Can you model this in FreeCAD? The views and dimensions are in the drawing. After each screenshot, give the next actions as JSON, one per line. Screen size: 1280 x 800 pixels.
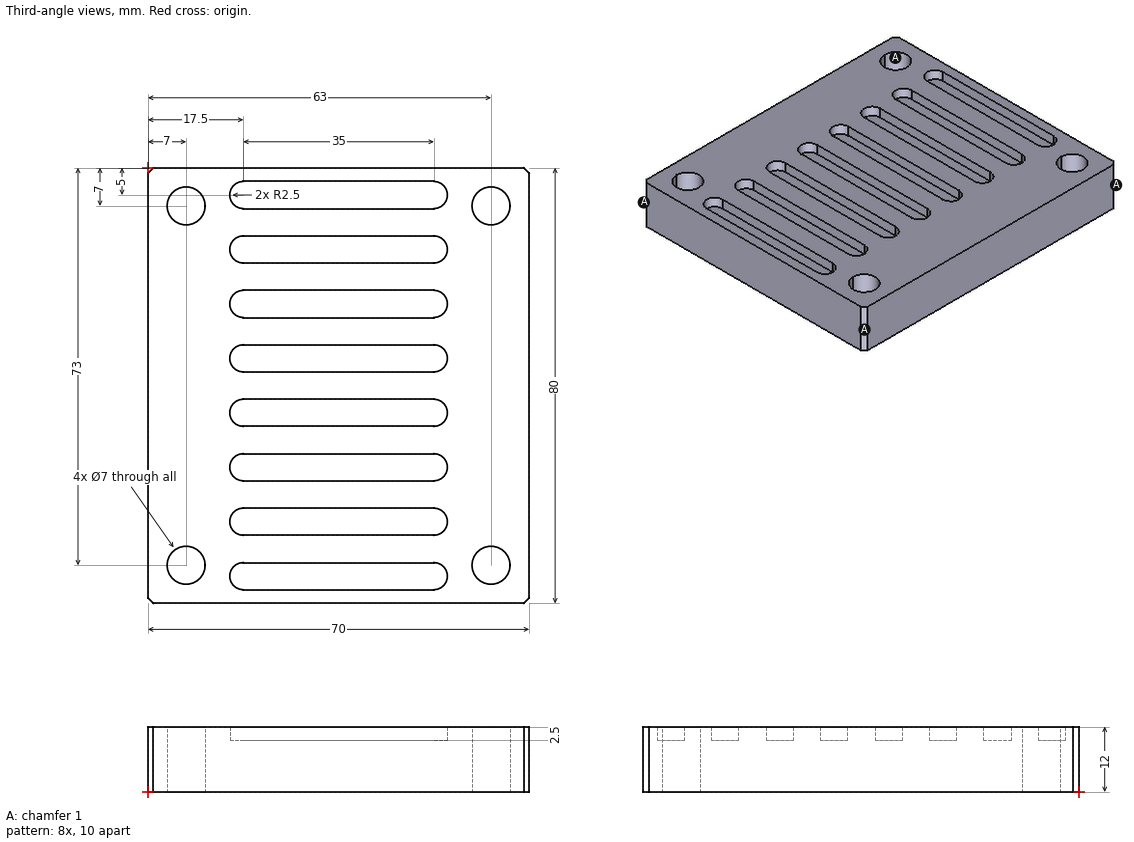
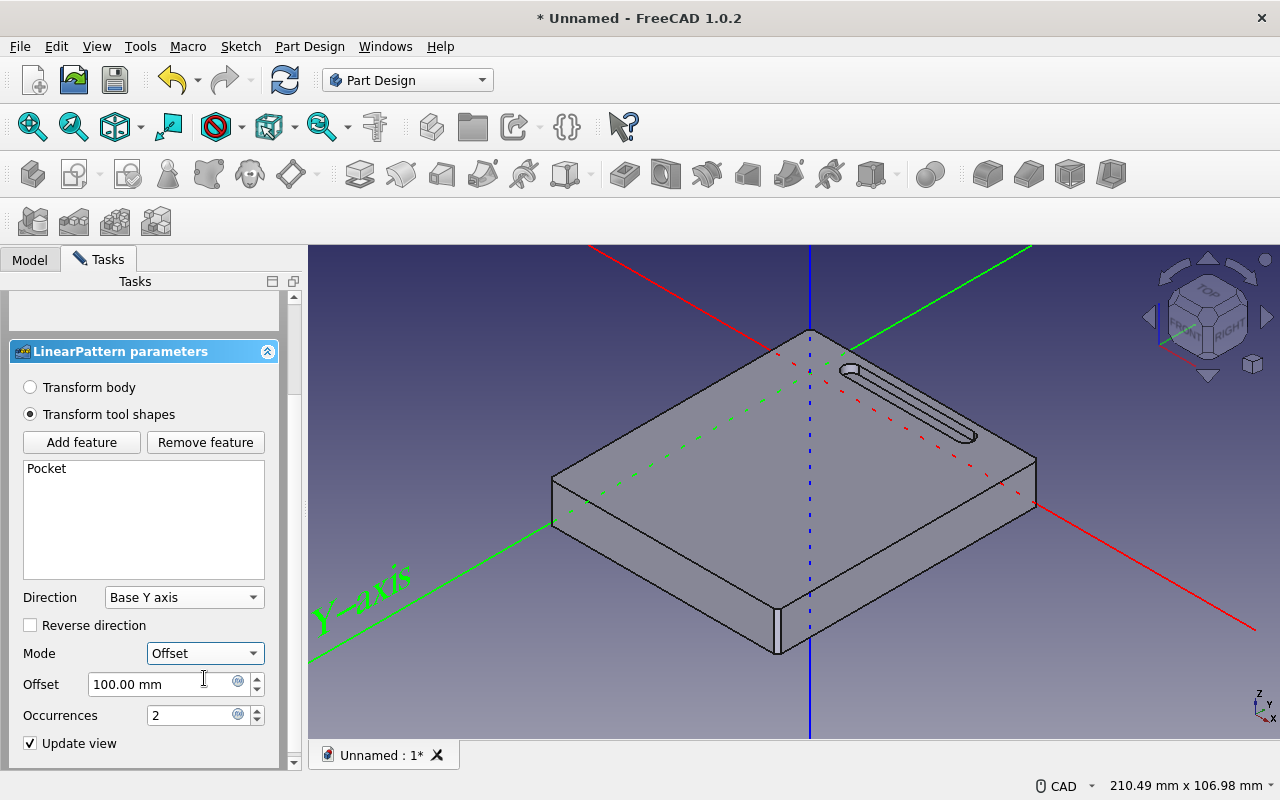
{"action": "triple_click", "coordinate": [170, 684]}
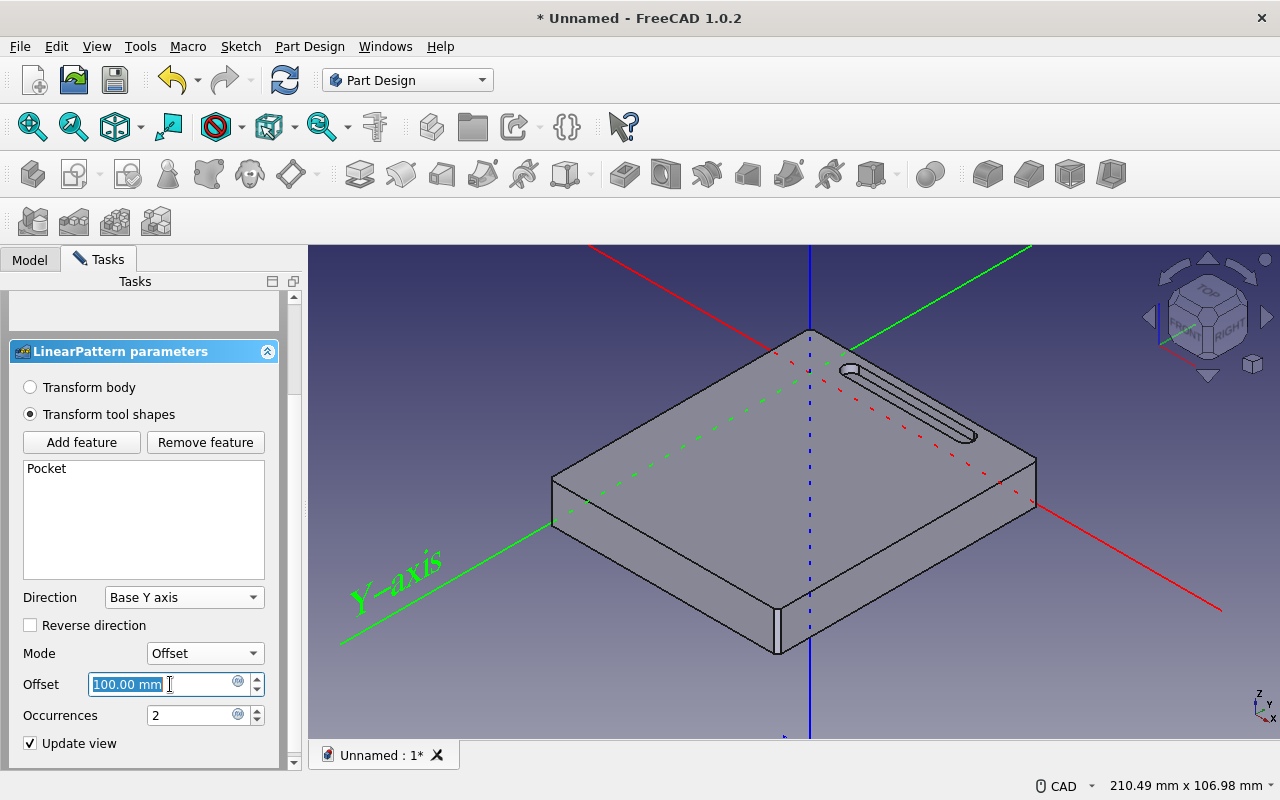
{"action": "type", "text": "10"}
{"action": "key", "text": "Tab"}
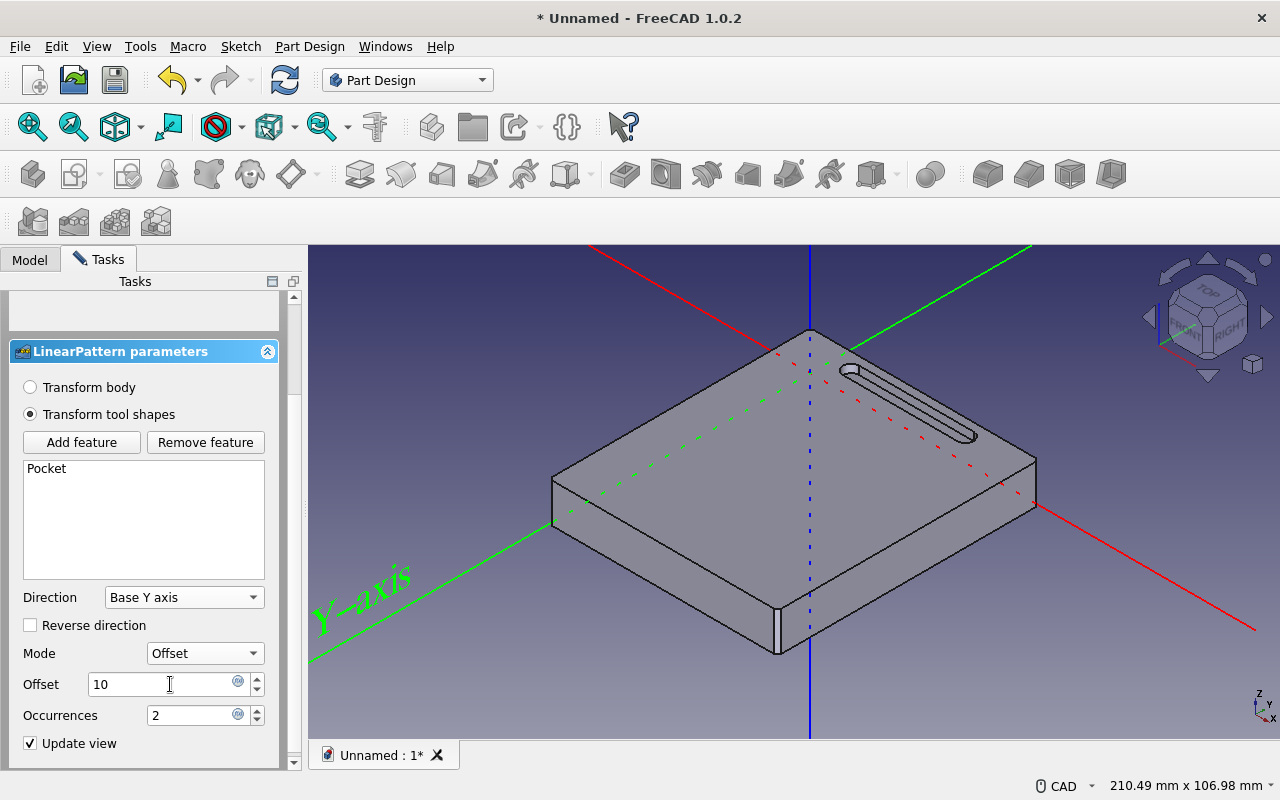
{"action": "triple_click", "coordinate": [199, 716]}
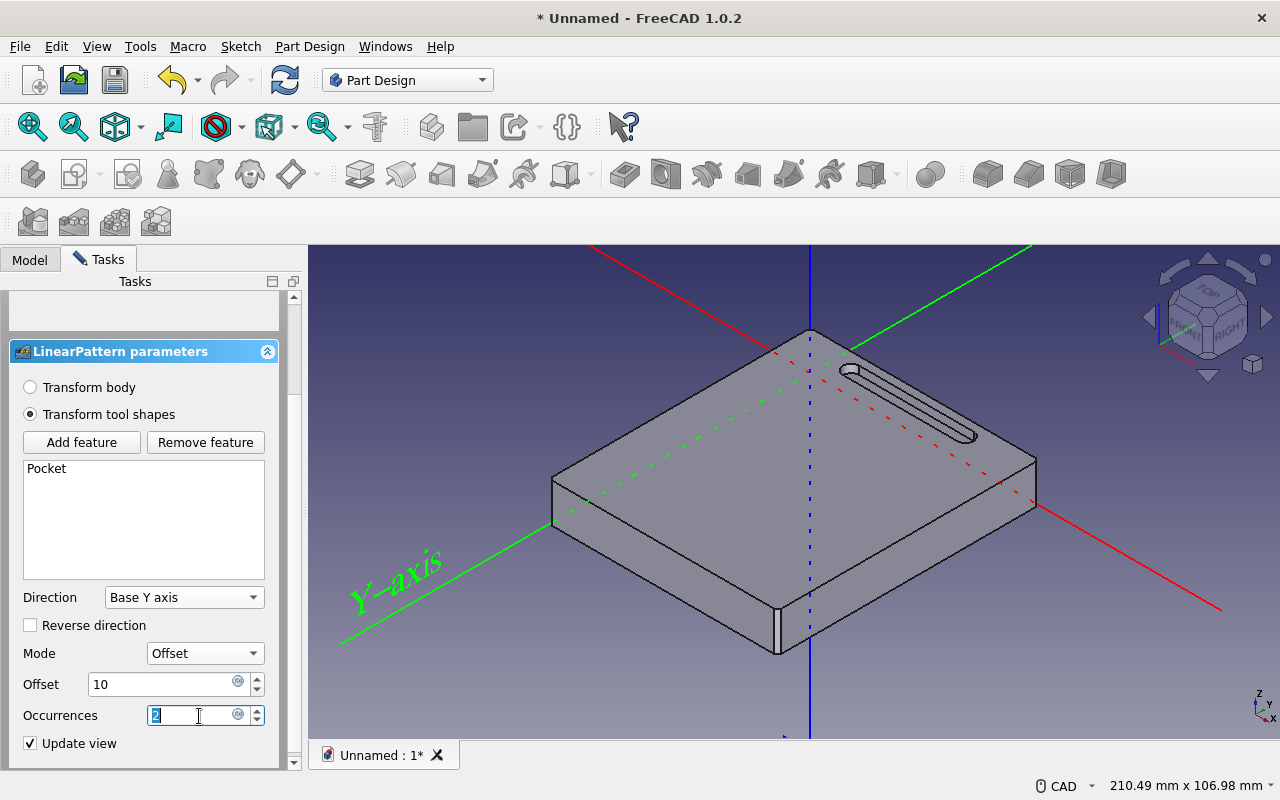
{"action": "type", "text": "8"}
{"action": "key", "text": "Tab"}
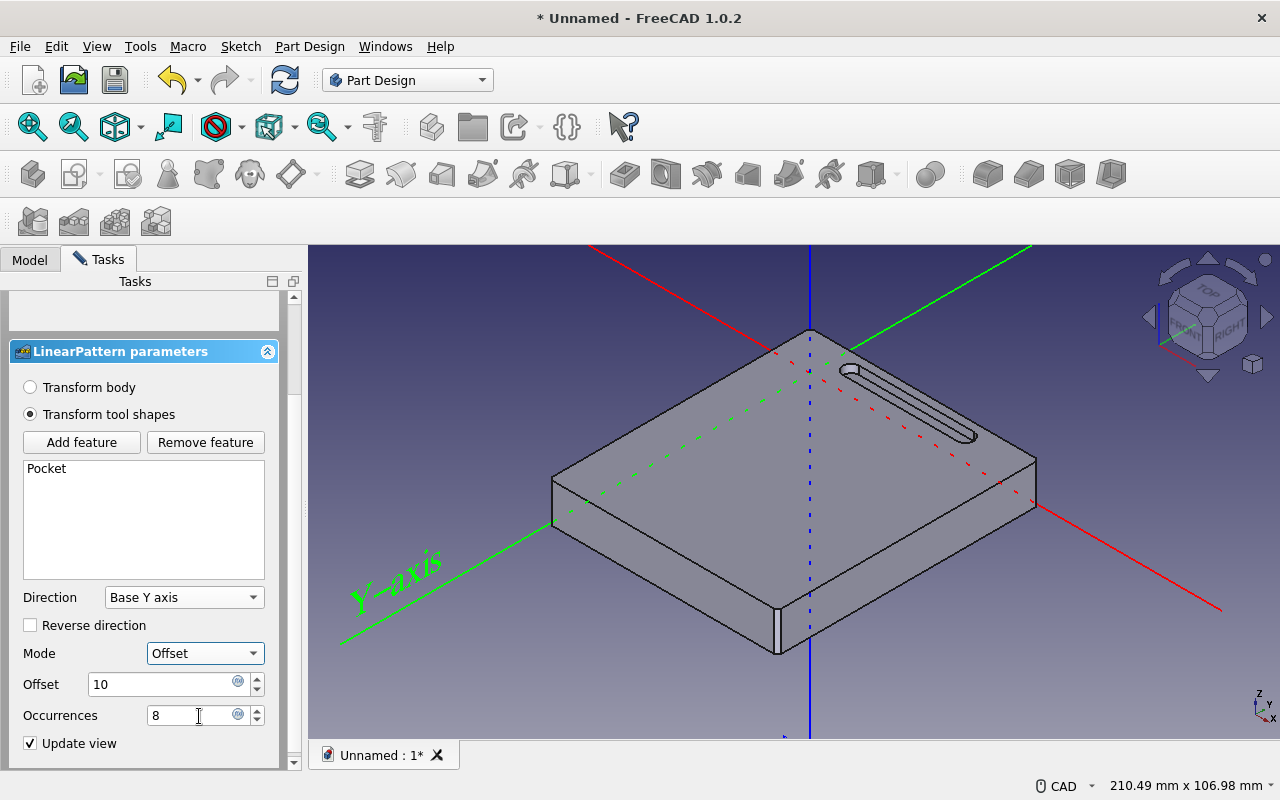
{"action": "left_click", "coordinate": [31, 625]}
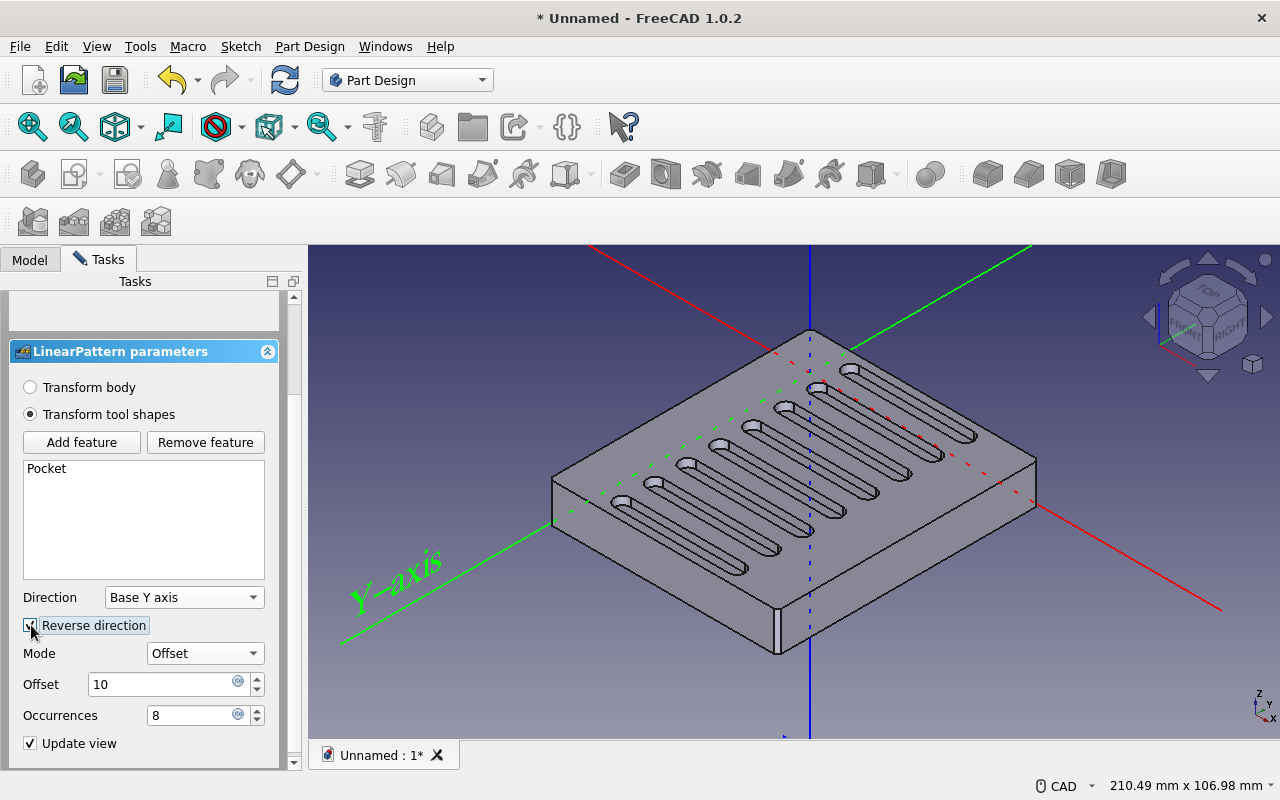
{"action": "scroll", "coordinate": [294, 530], "scroll_direction": "up", "scroll_amount": 3}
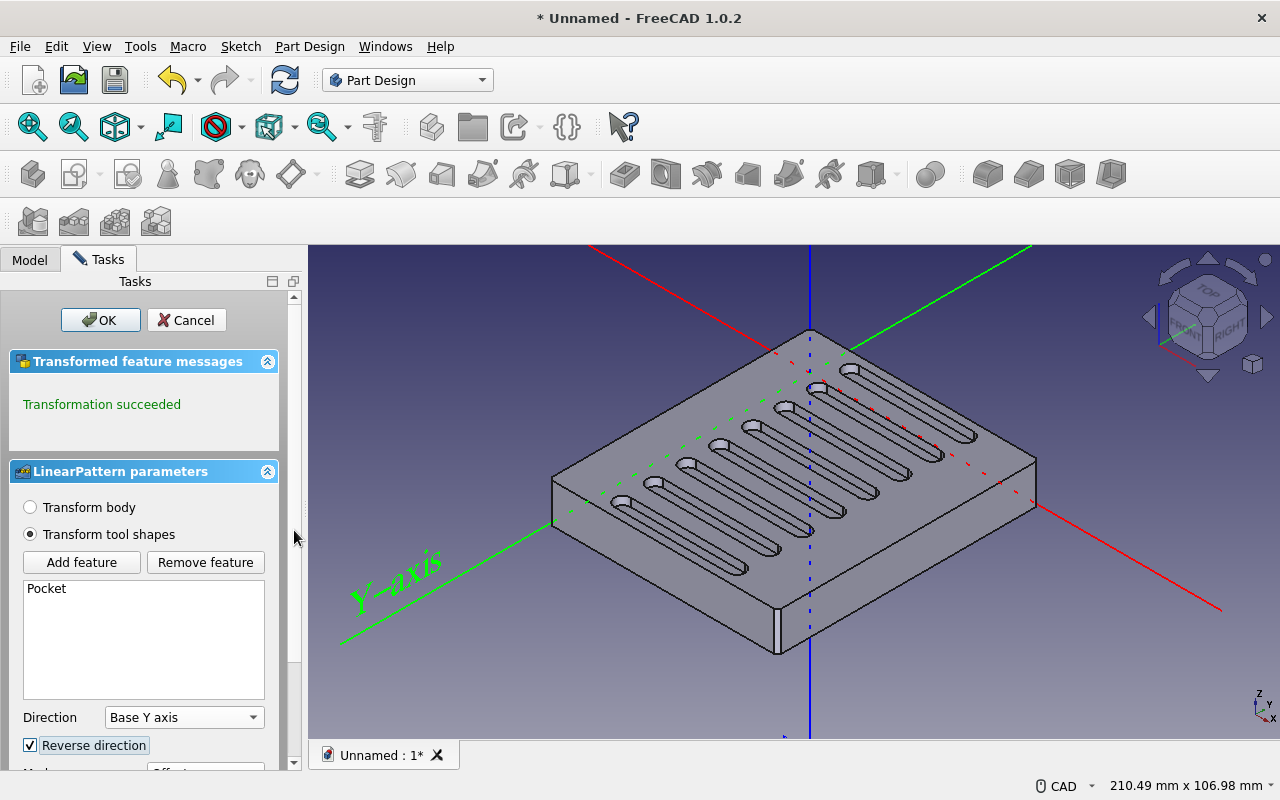
{"action": "left_click", "coordinate": [101, 320]}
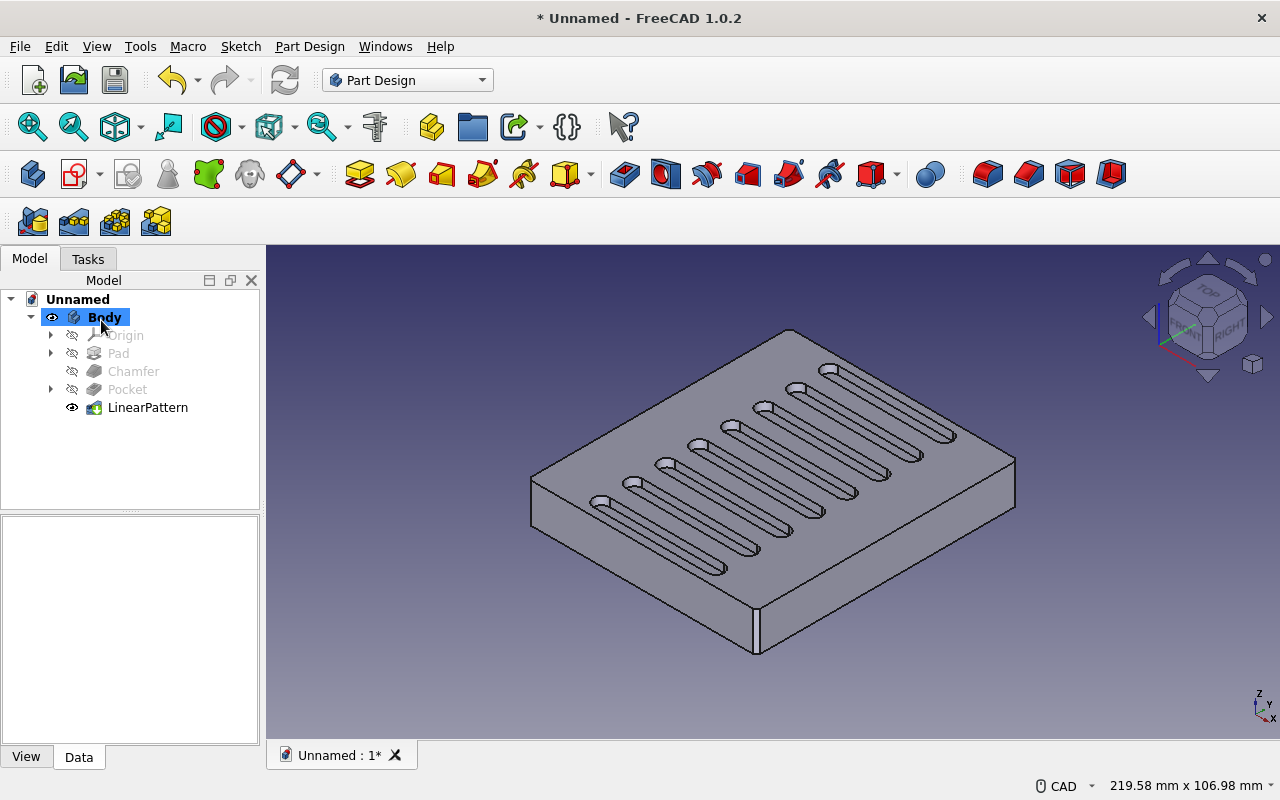
{"action": "left_click", "coordinate": [74, 174]}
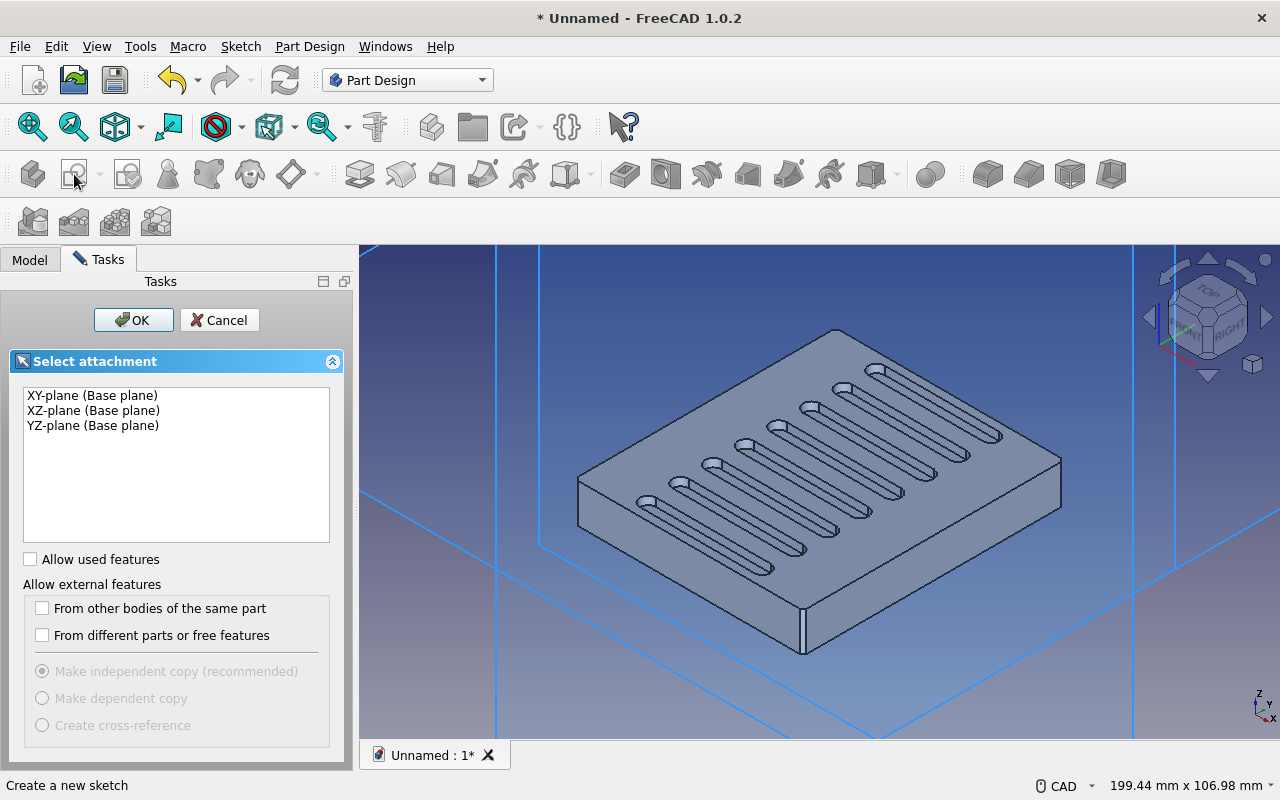
{"action": "left_click", "coordinate": [84, 396]}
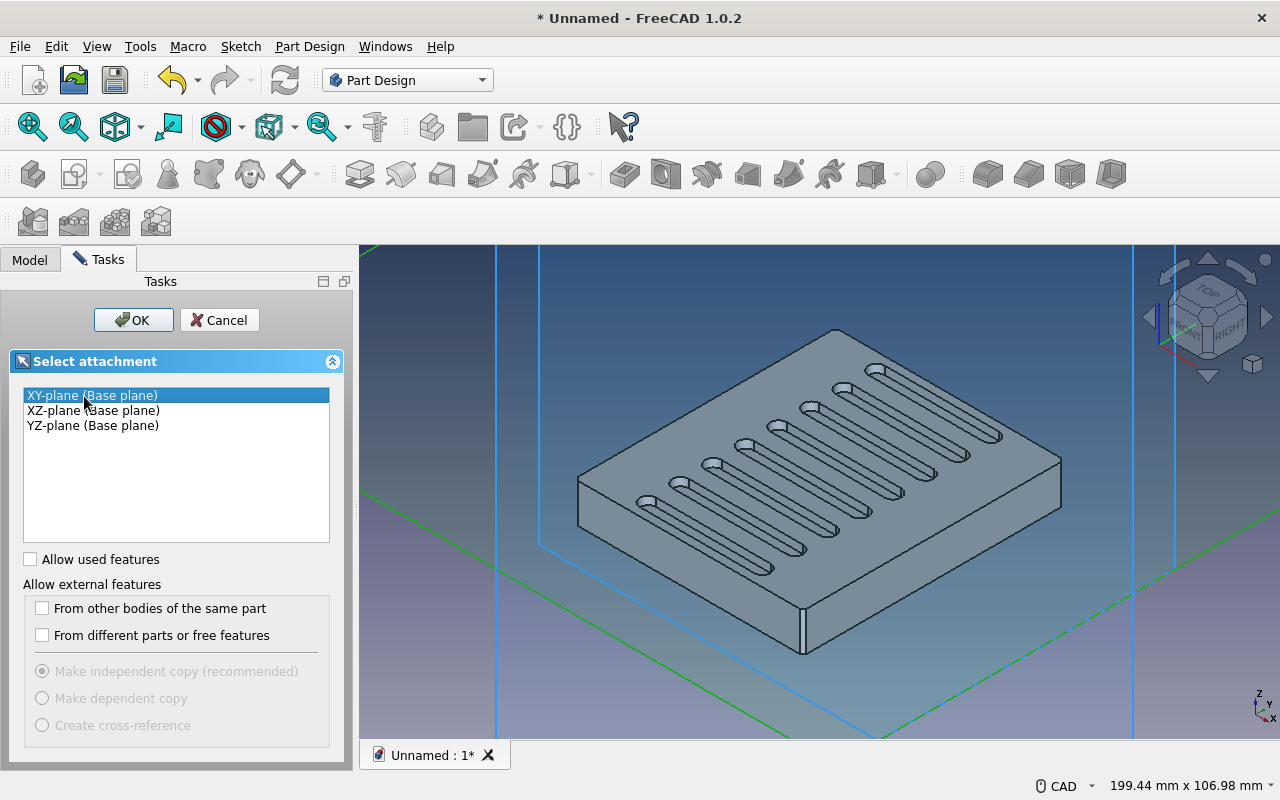
{"action": "left_click", "coordinate": [134, 320]}